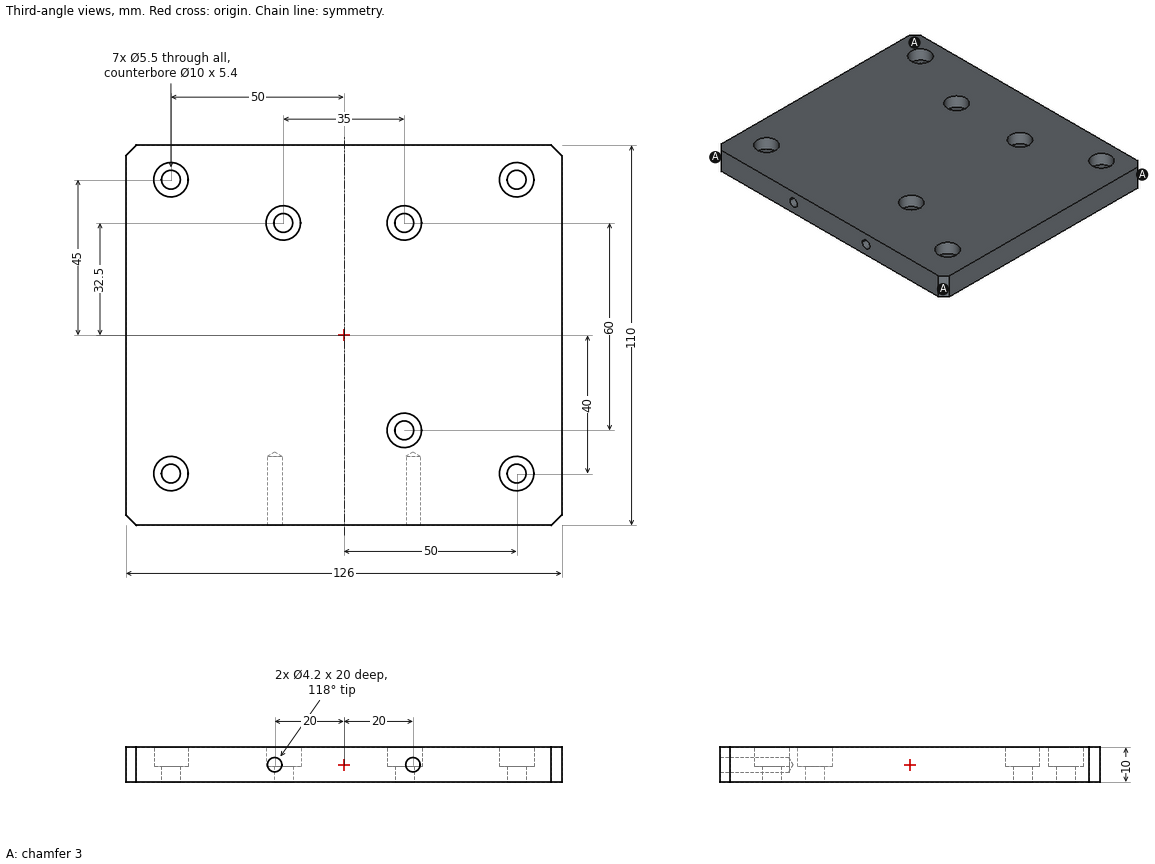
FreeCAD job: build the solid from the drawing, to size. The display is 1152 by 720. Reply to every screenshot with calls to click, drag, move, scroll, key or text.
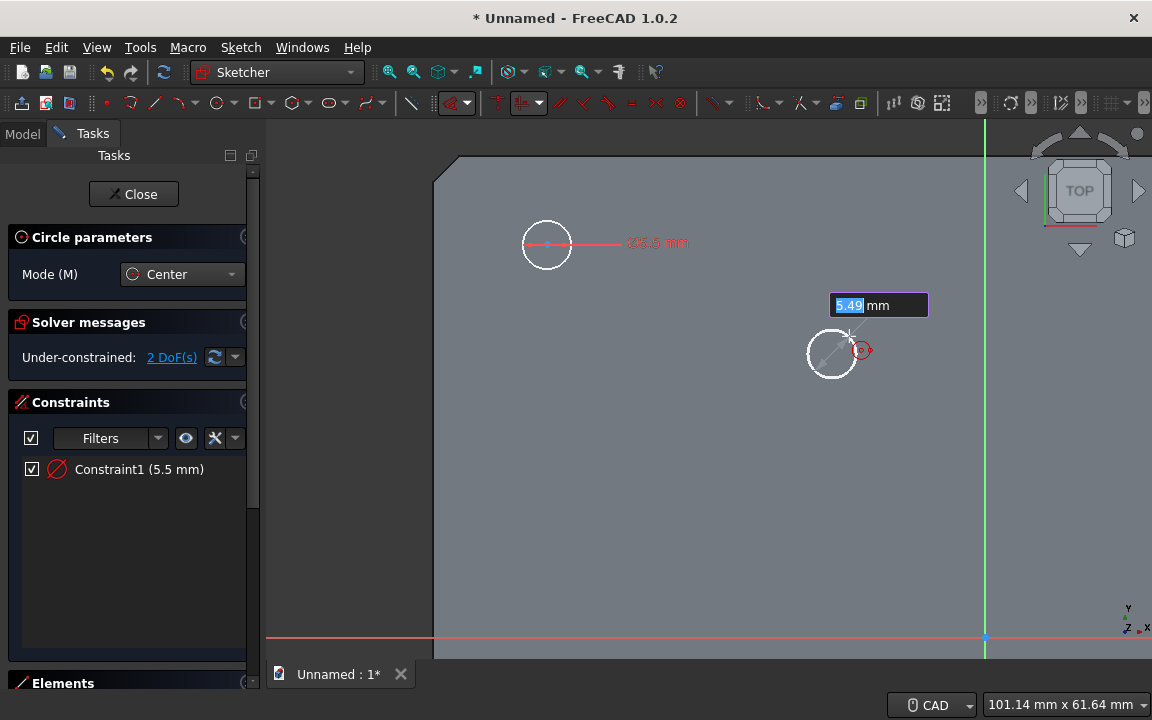
text(5.5)
key(Return)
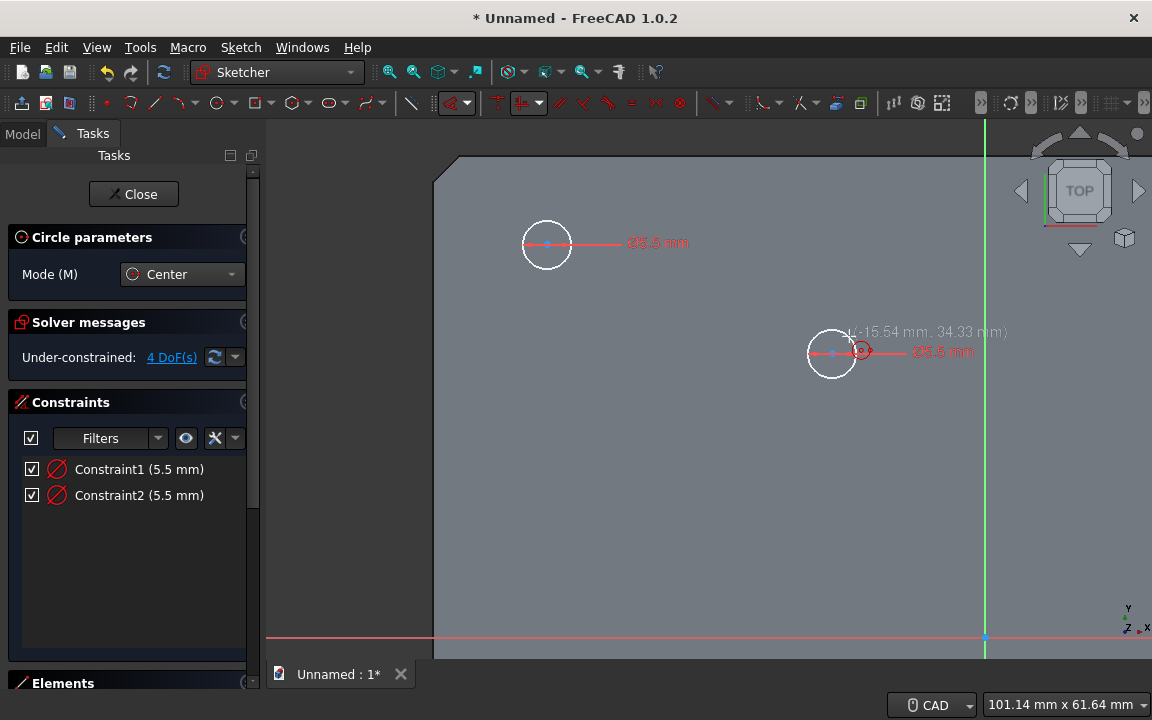
scroll(359, 204, down, 4)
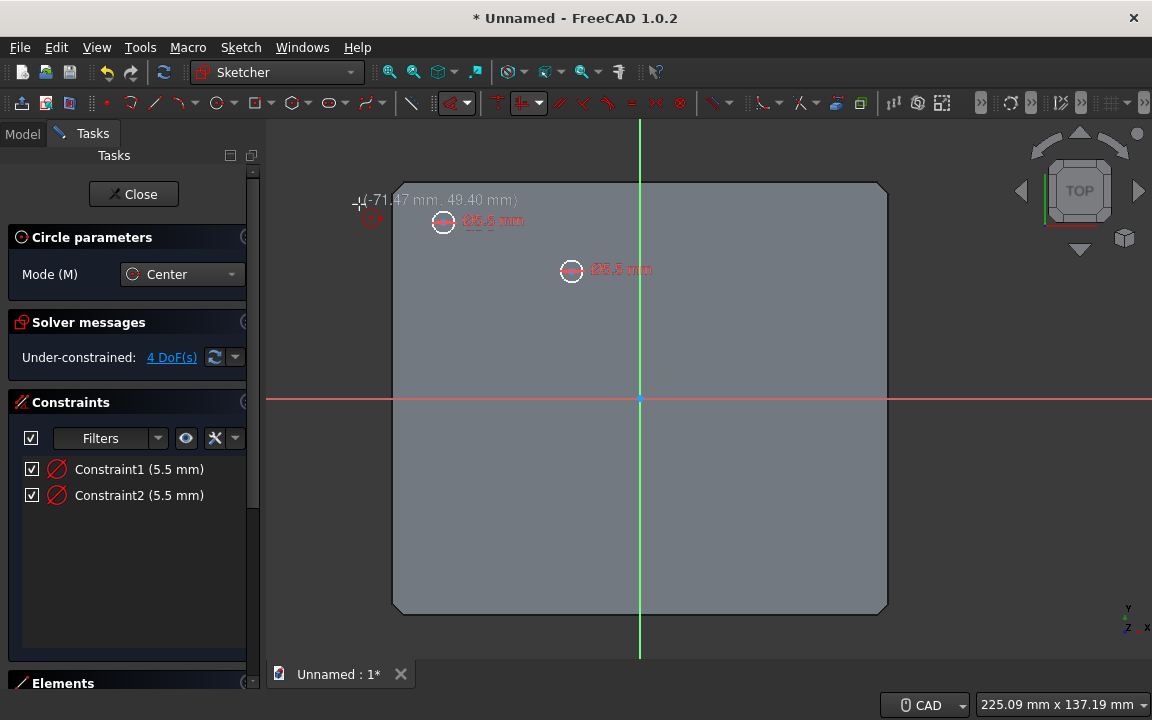
scroll(709, 271, up, 4)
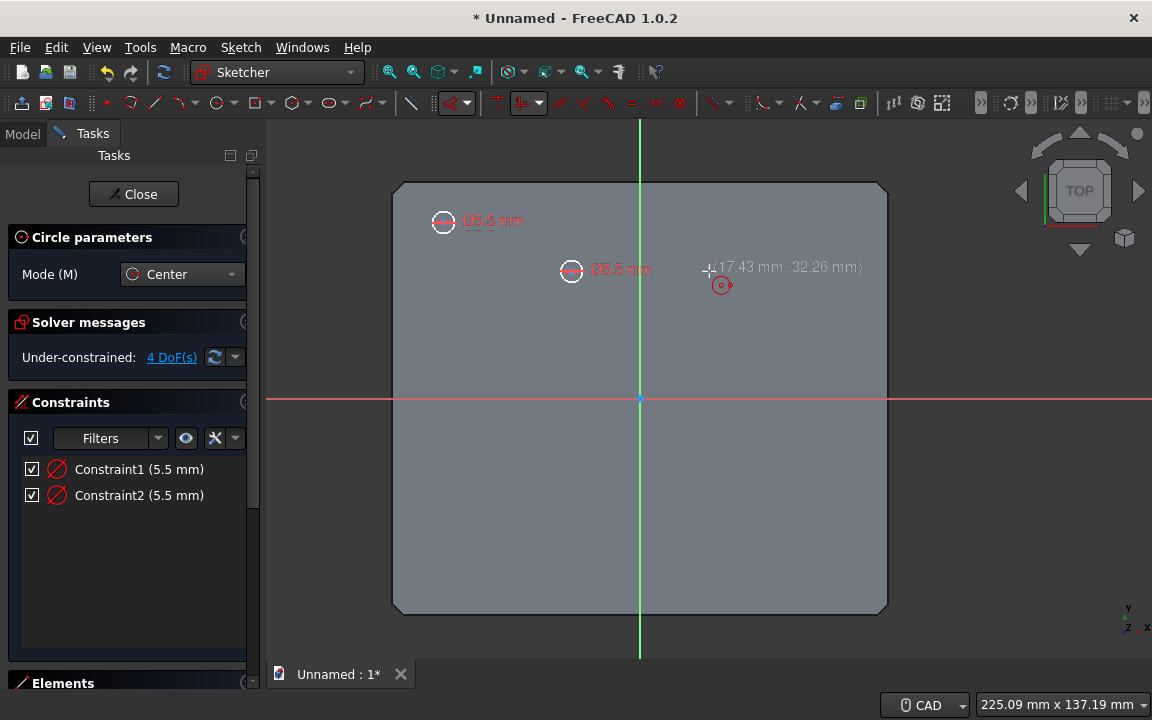
click(709, 271)
move(726, 254)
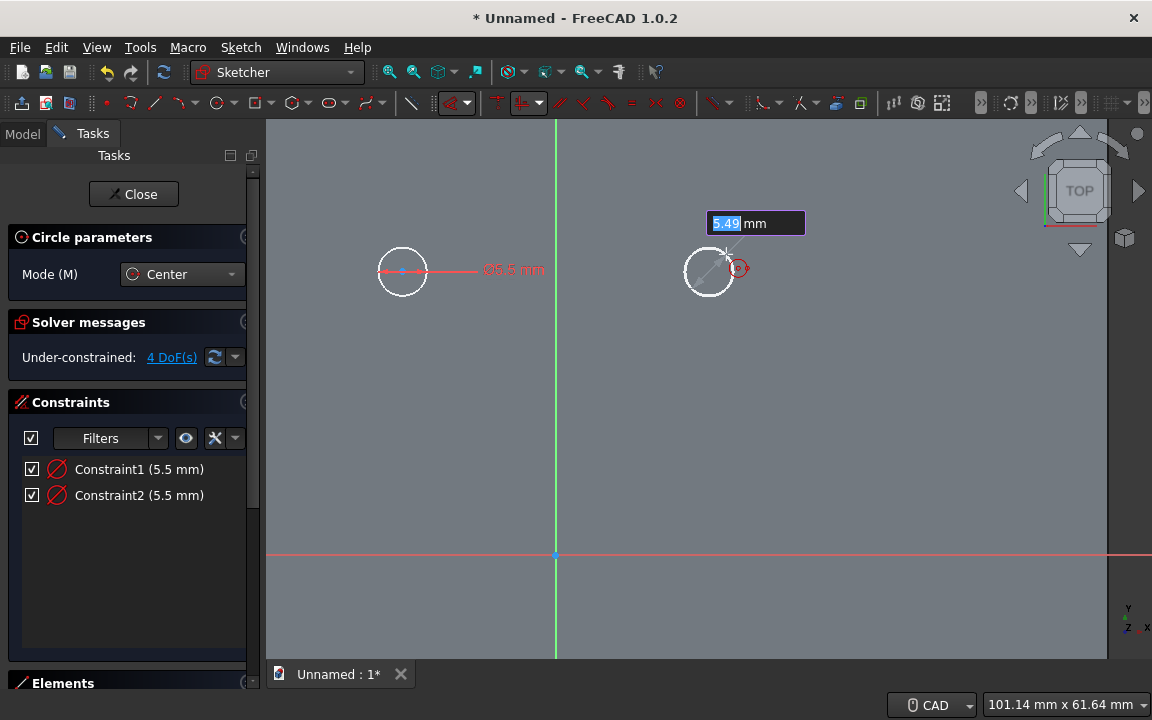
text(5.5)
key(Return)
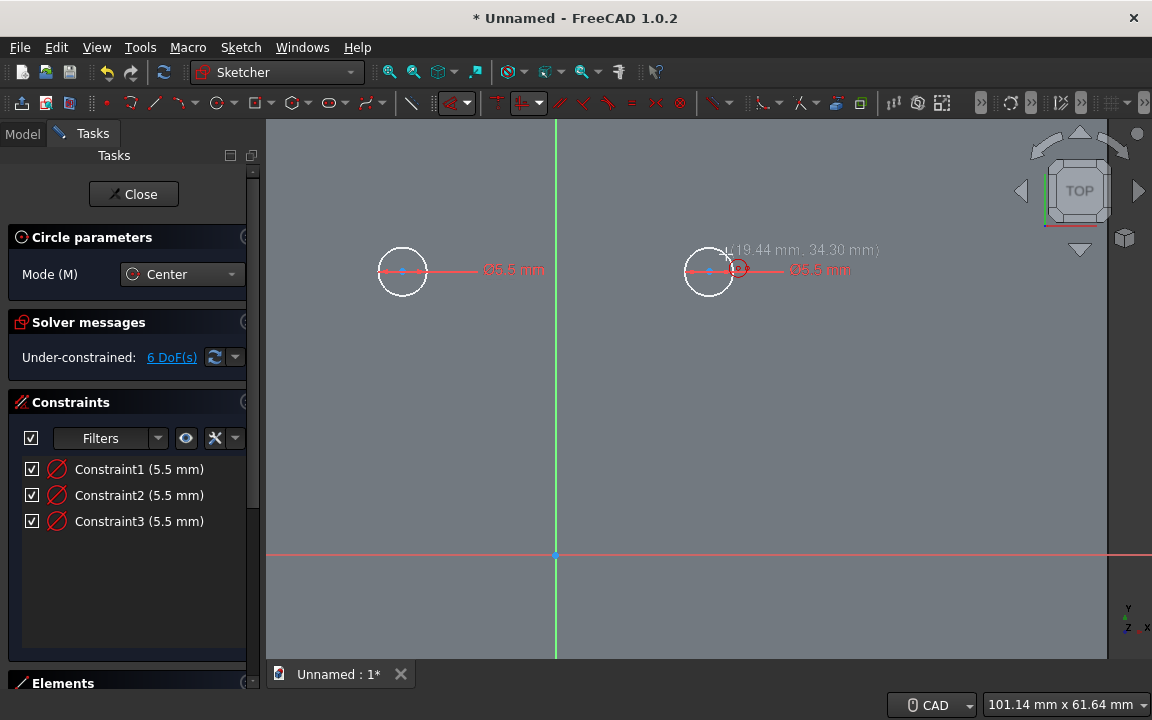
scroll(710, 271, down, 4)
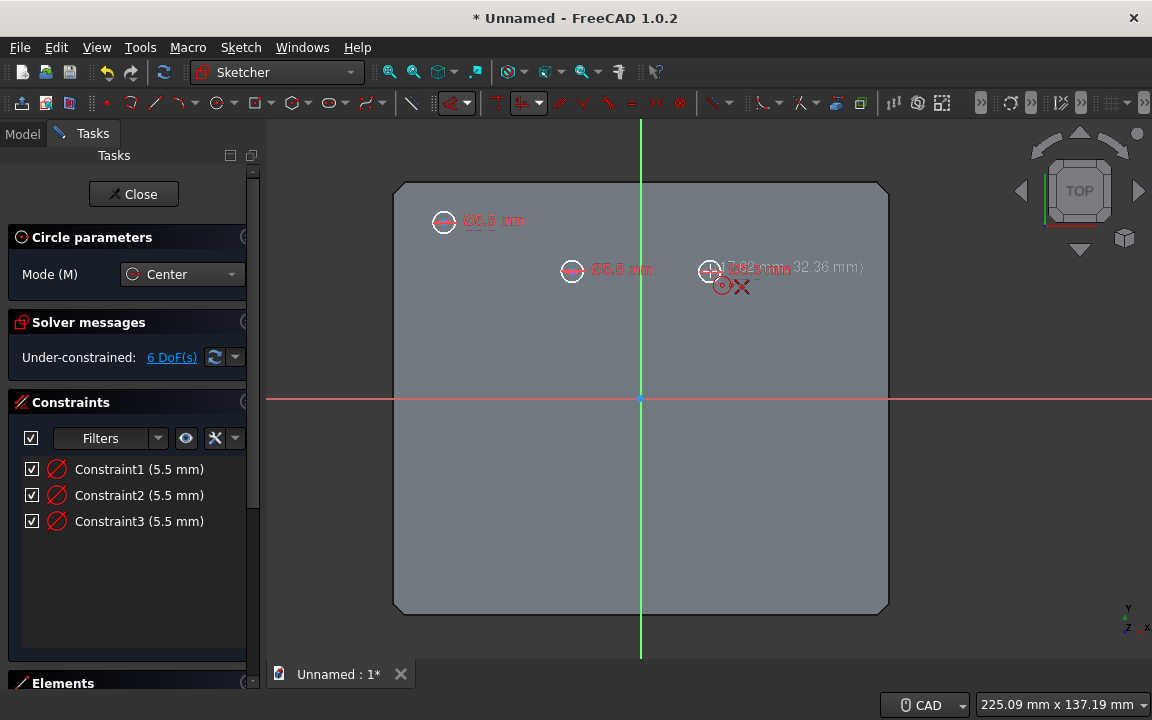
scroll(838, 222, up, 4)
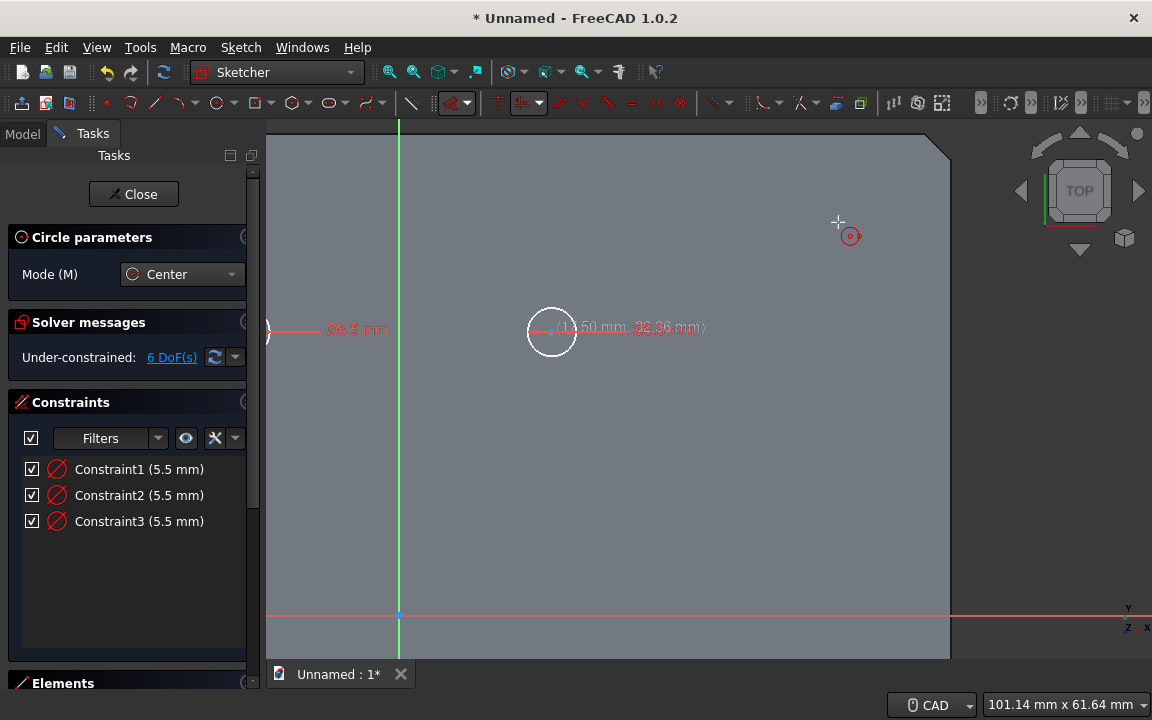
click(837, 221)
move(854, 204)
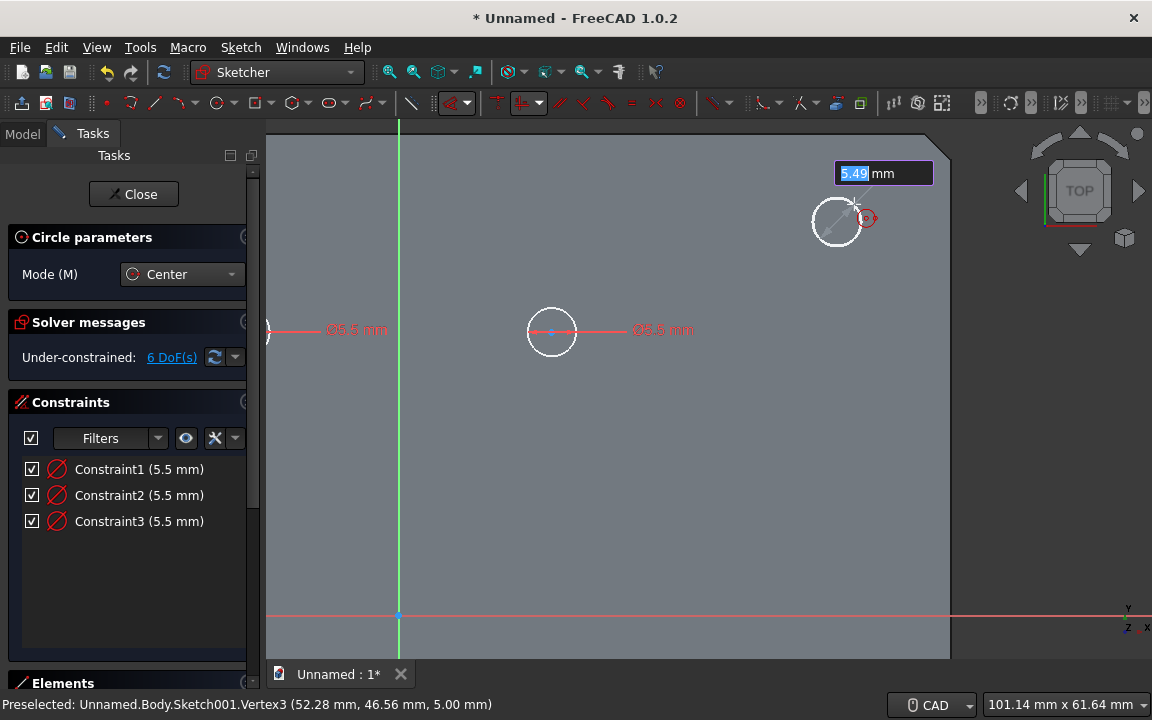
text(5.5)
key(Return)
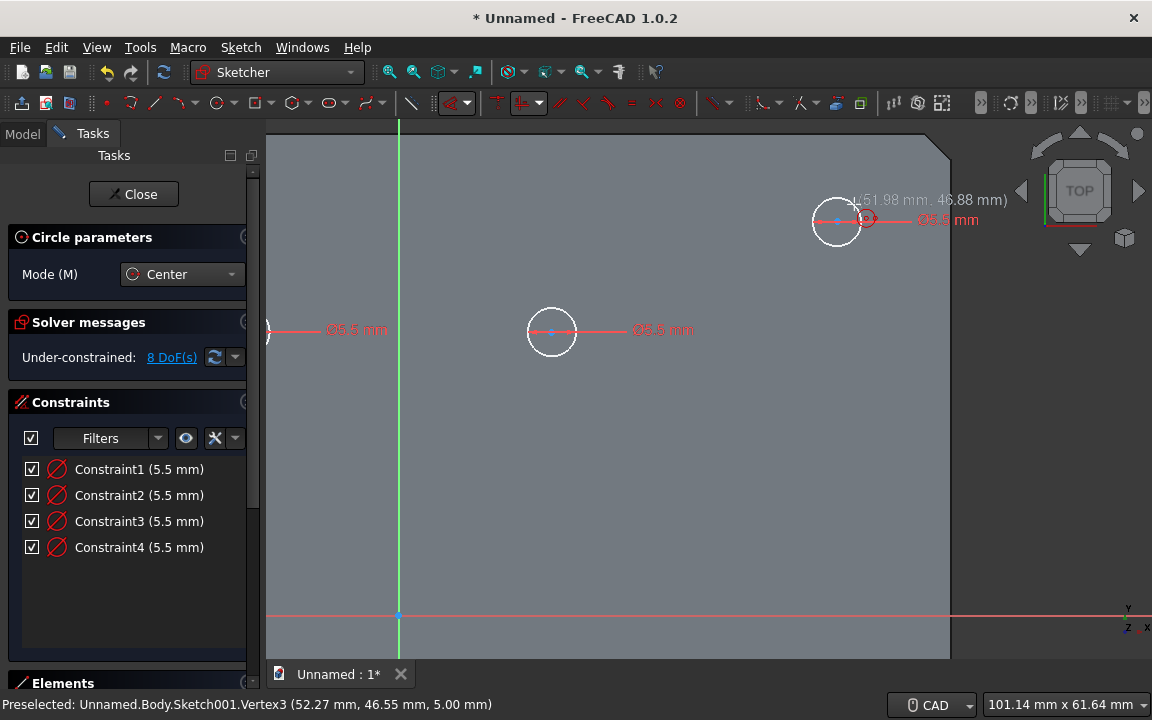
scroll(838, 222, down, 4)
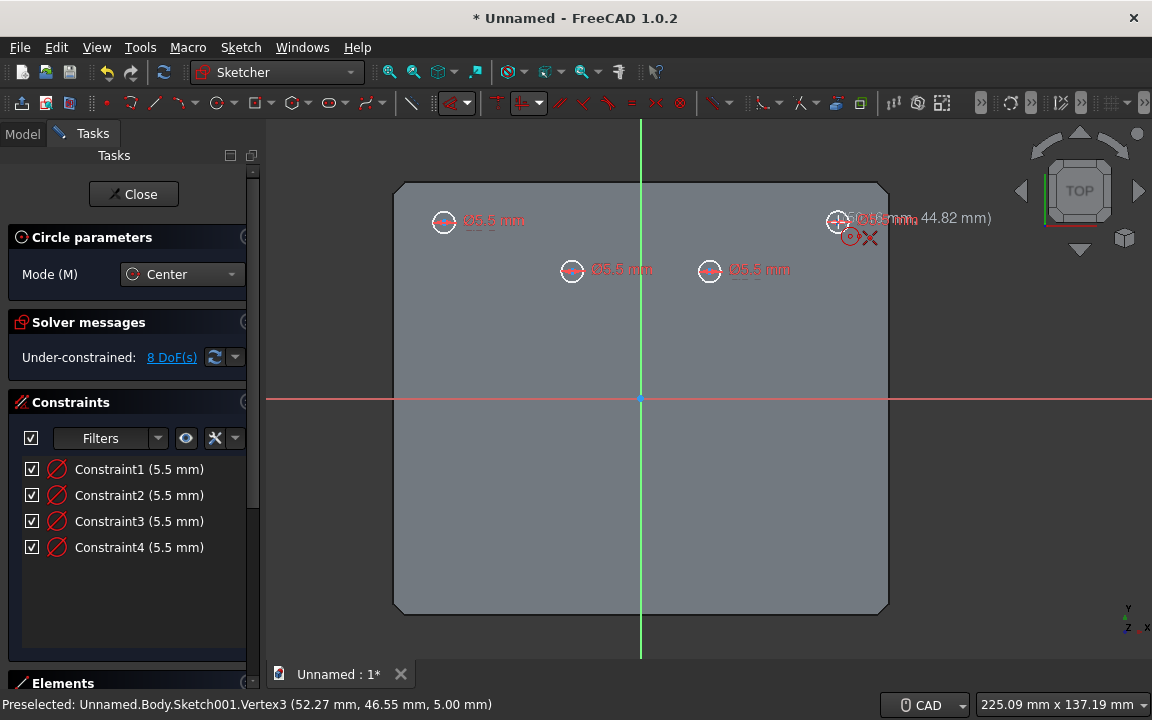
scroll(838, 556, up, 4)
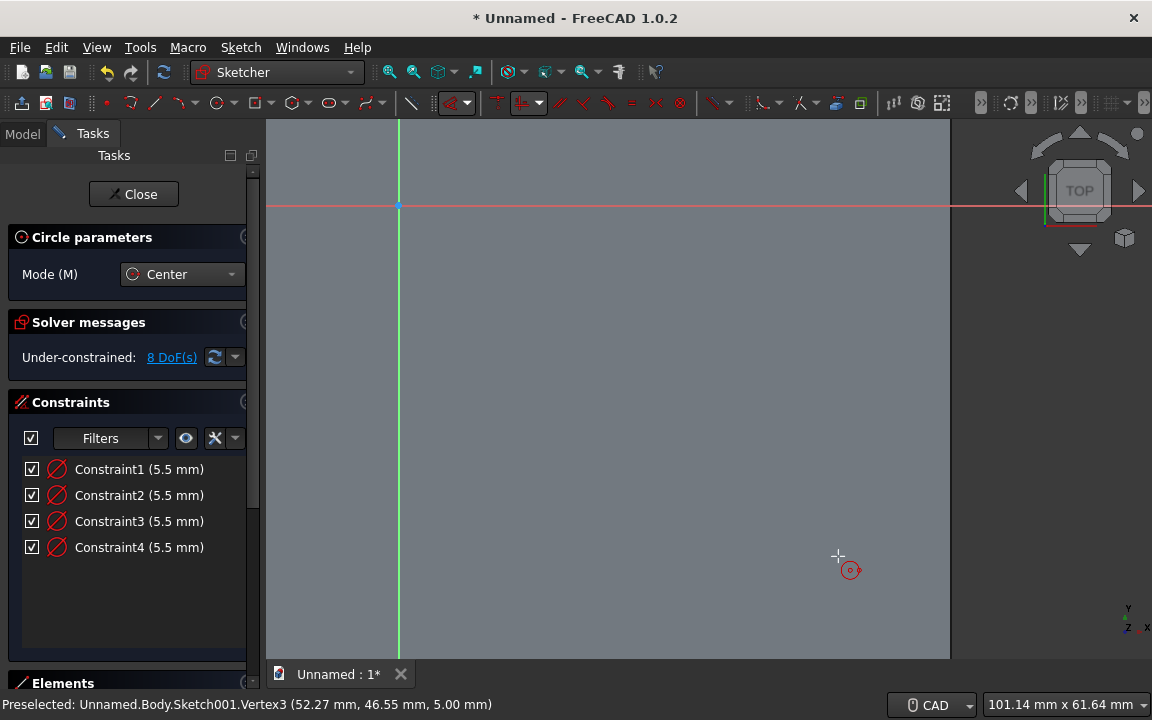
click(837, 556)
move(854, 539)